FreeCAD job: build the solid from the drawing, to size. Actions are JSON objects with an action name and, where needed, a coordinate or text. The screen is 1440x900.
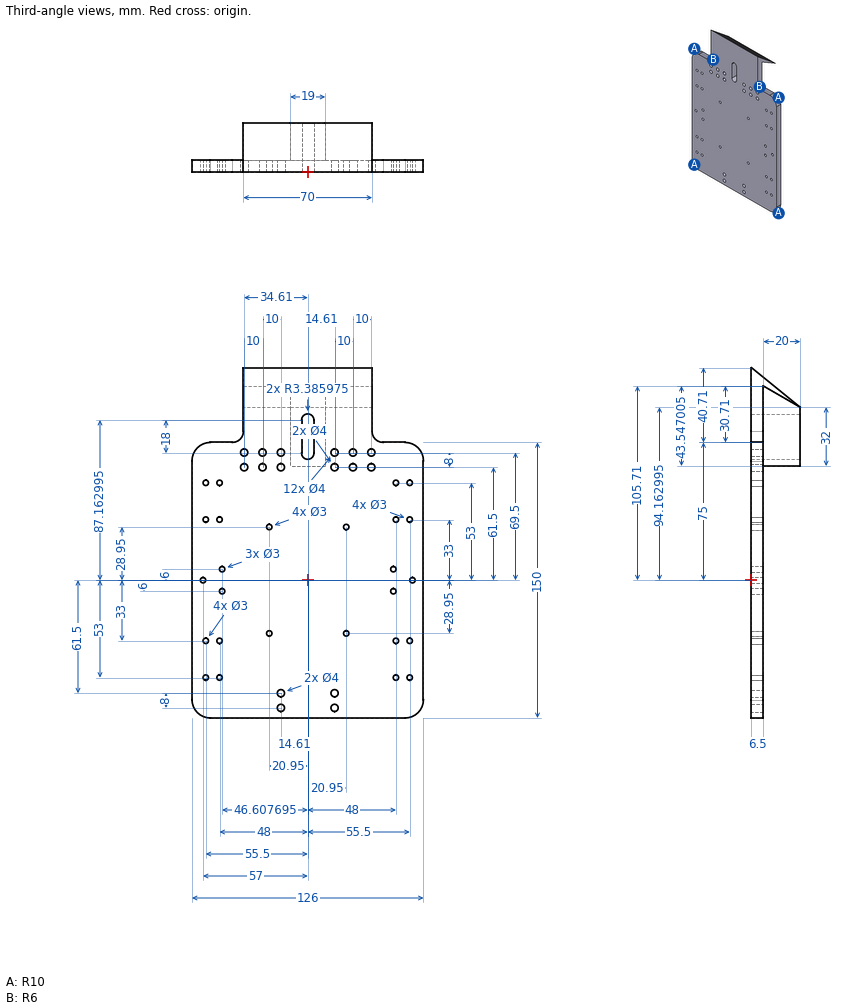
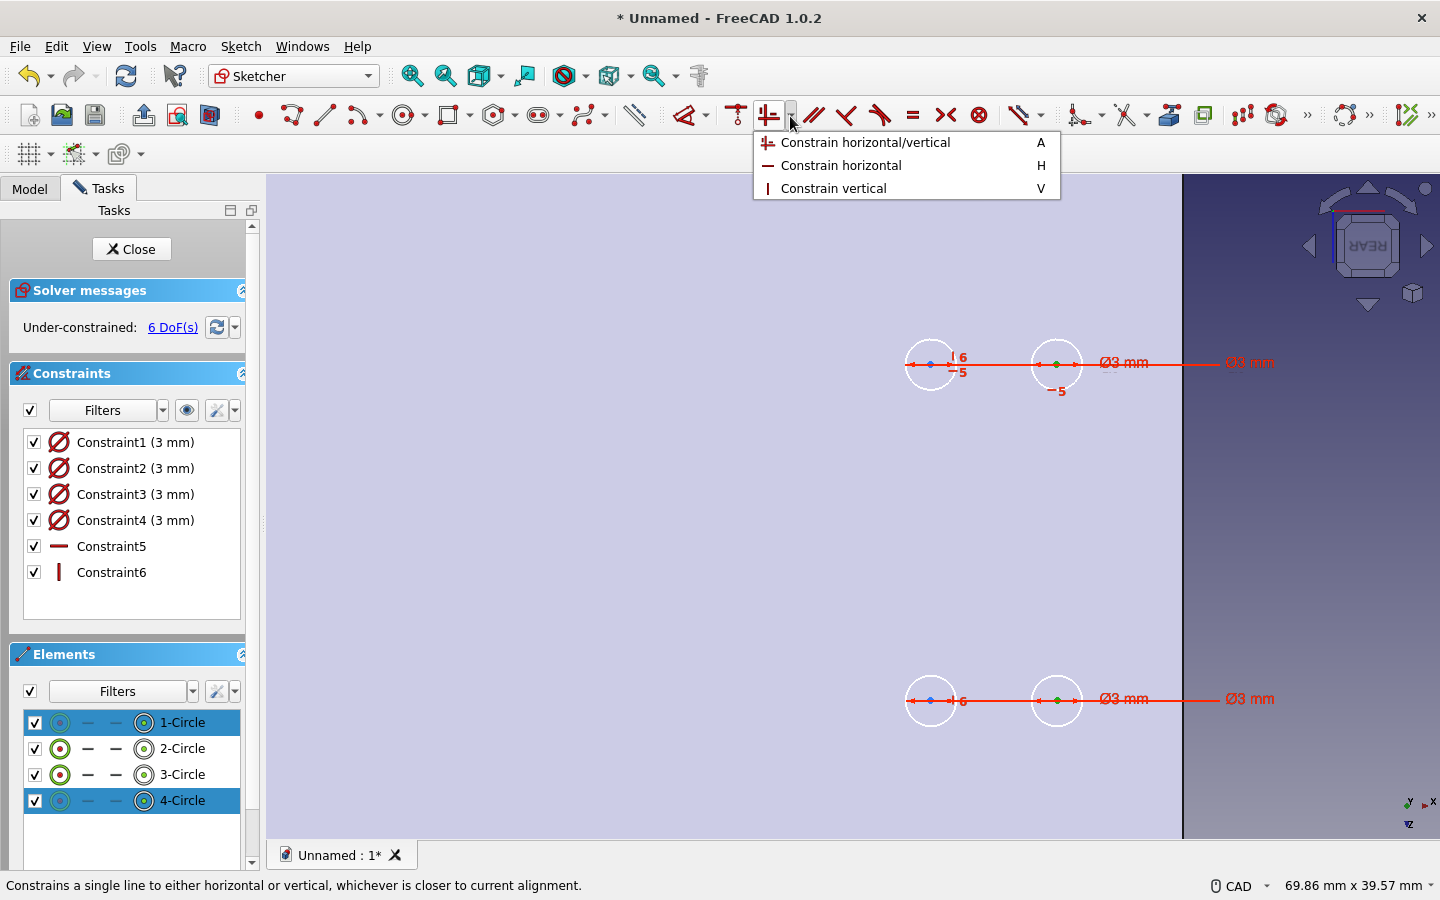
{"action": "left_click", "coordinate": [907, 188]}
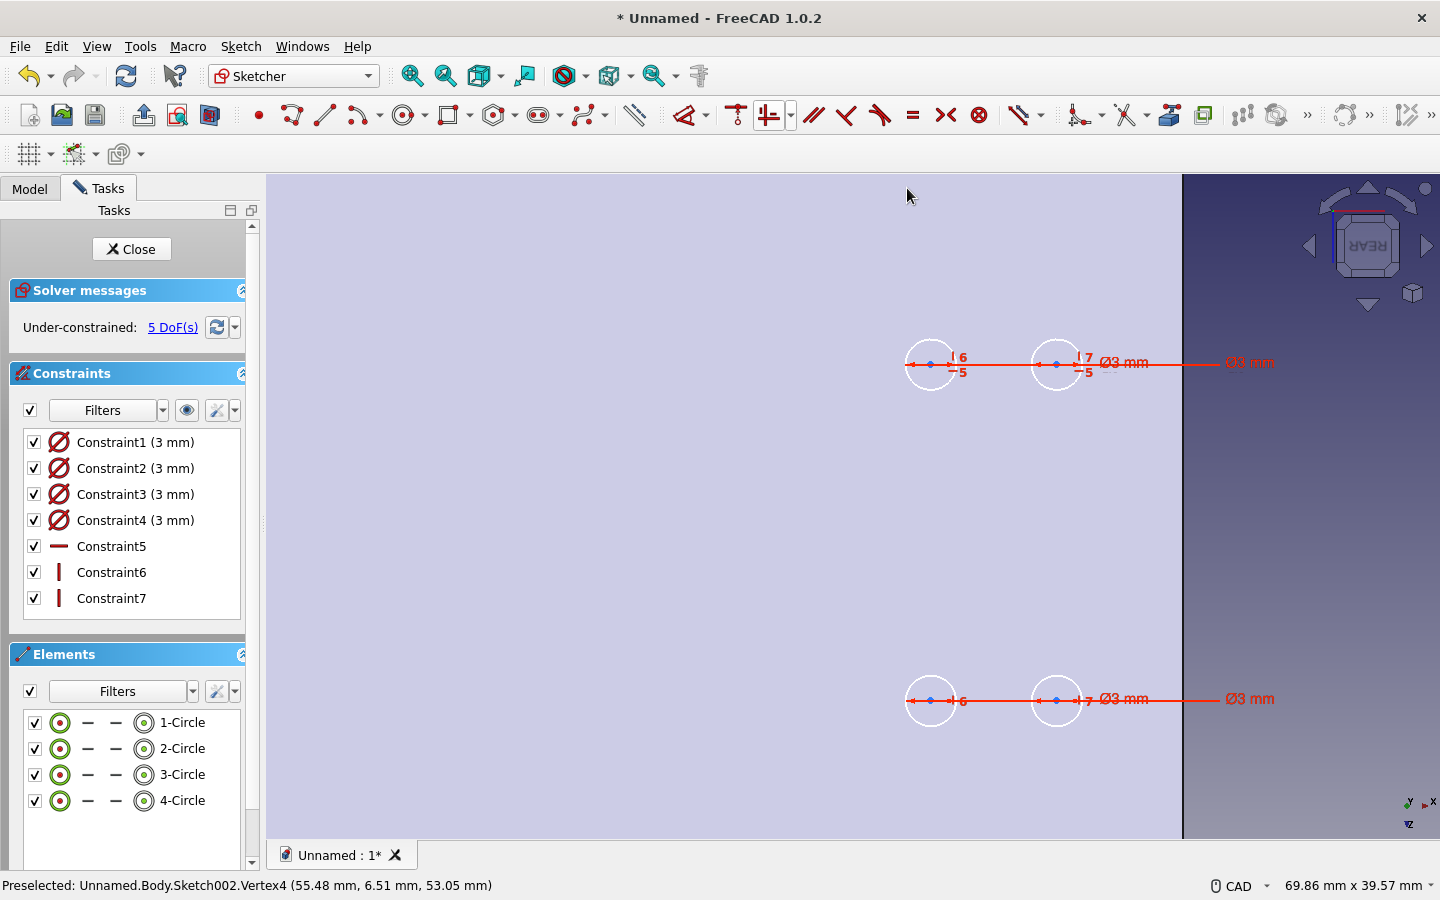
{"action": "left_click", "coordinate": [931, 701]}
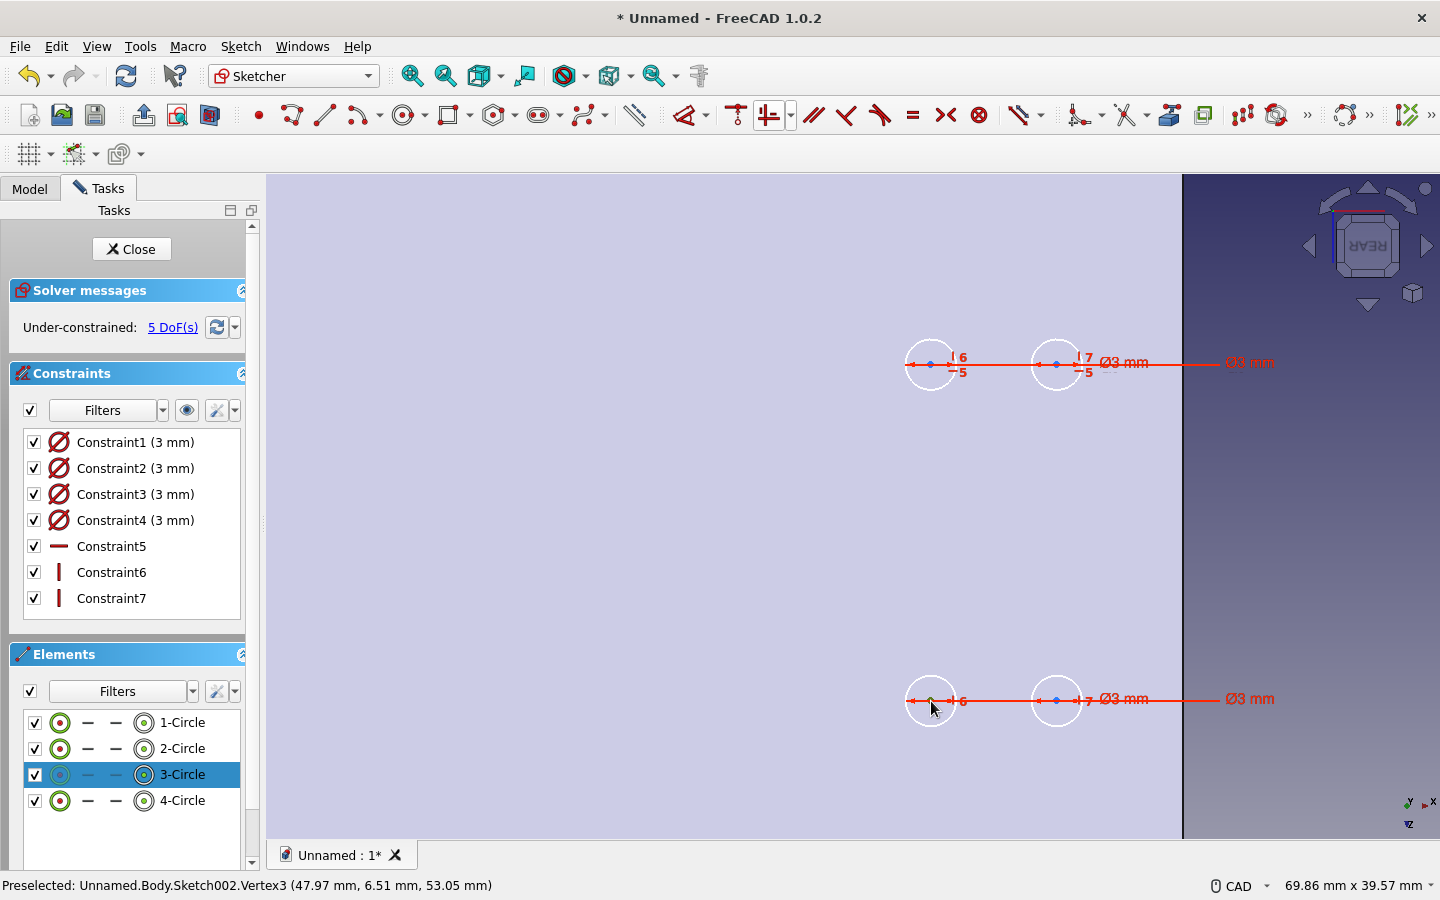
{"action": "left_click", "coordinate": [1057, 701]}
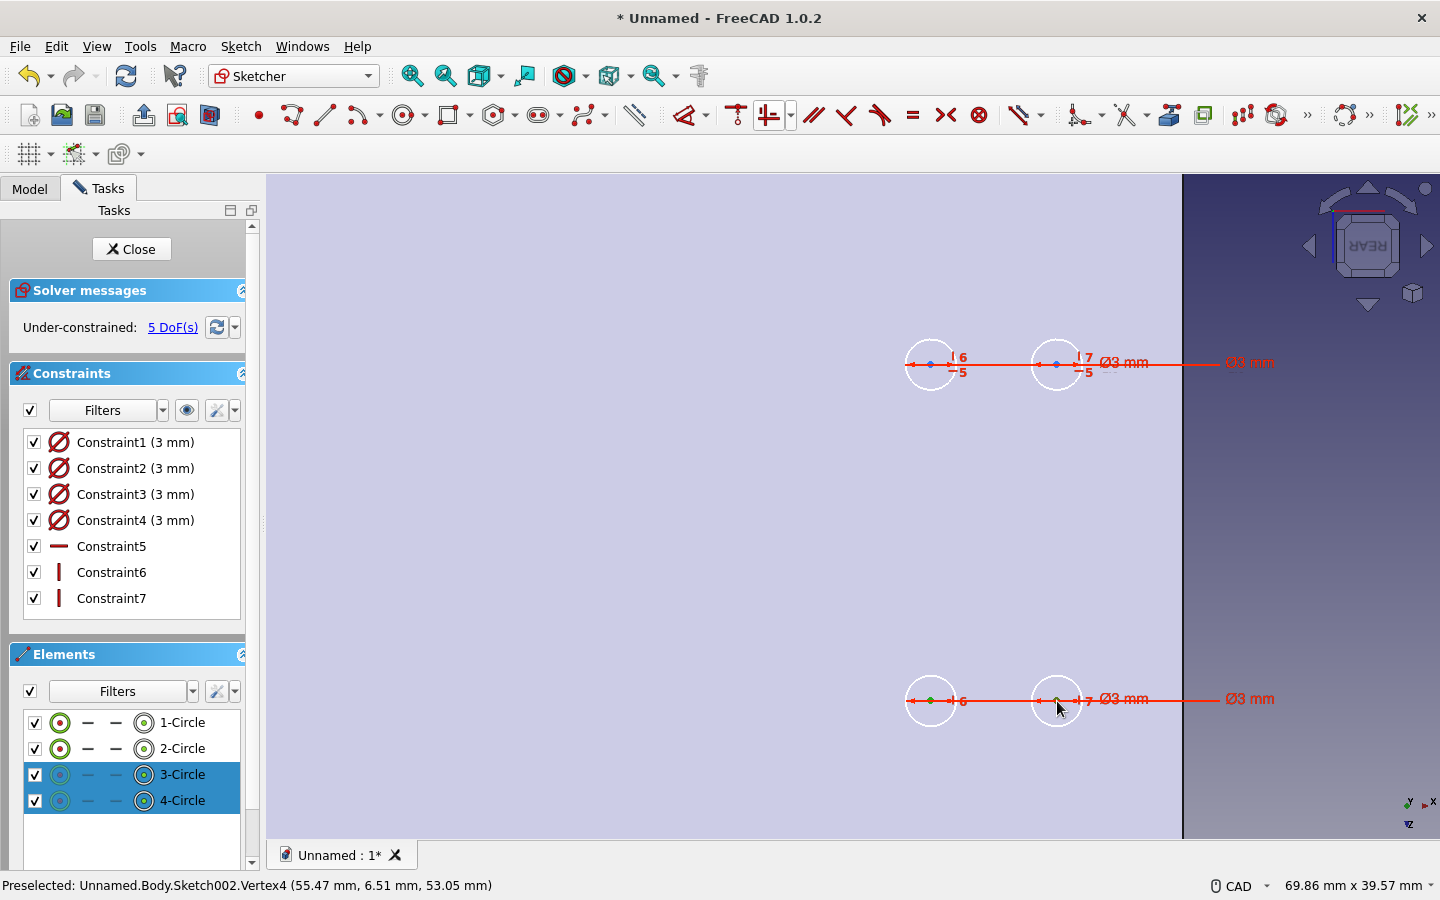
{"action": "key", "text": "h"}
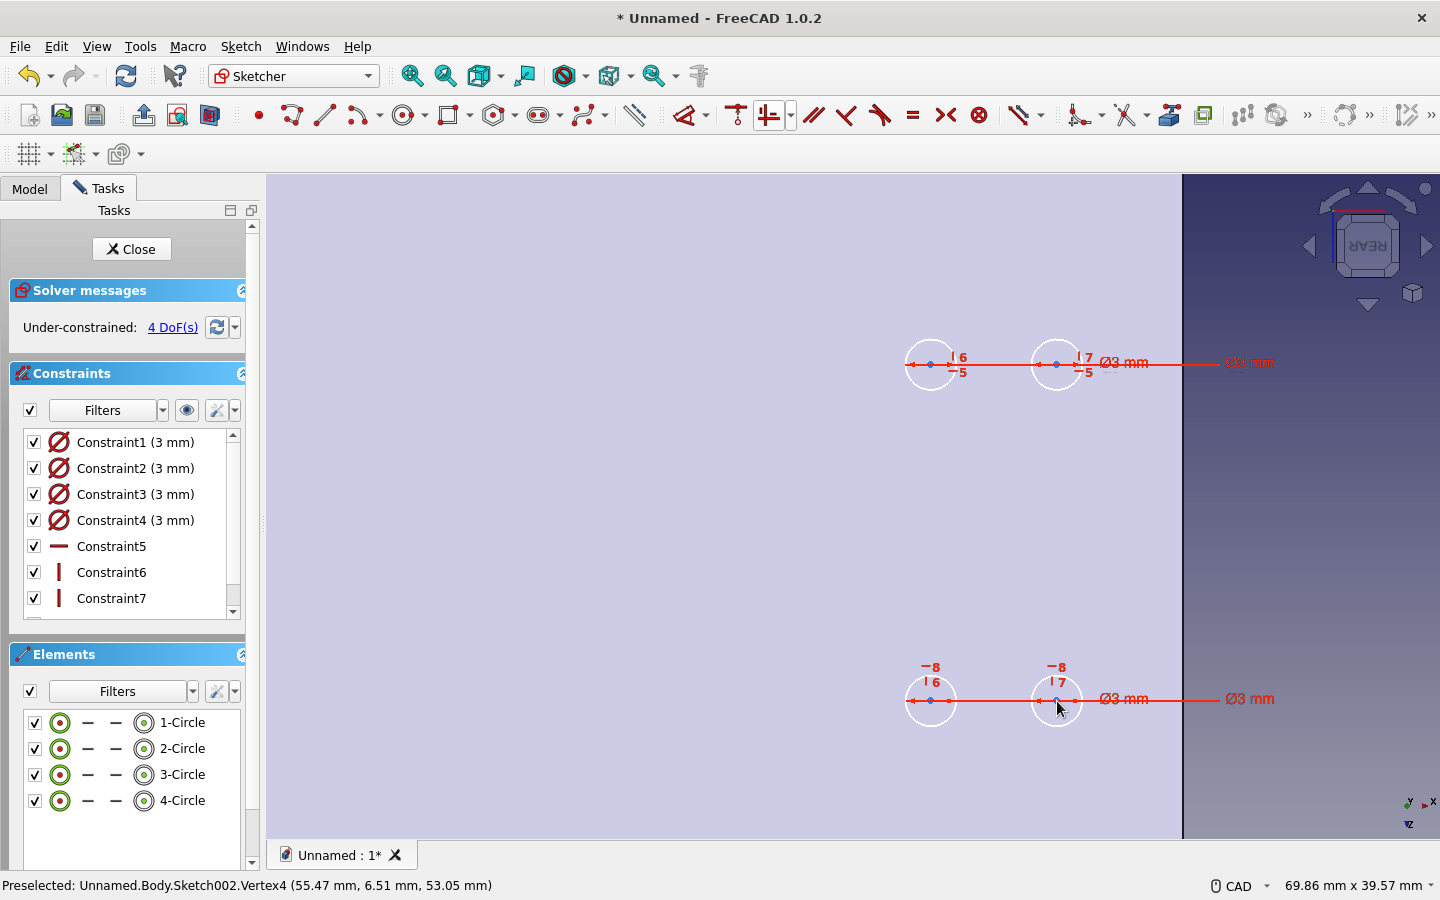
{"action": "key", "text": "d"}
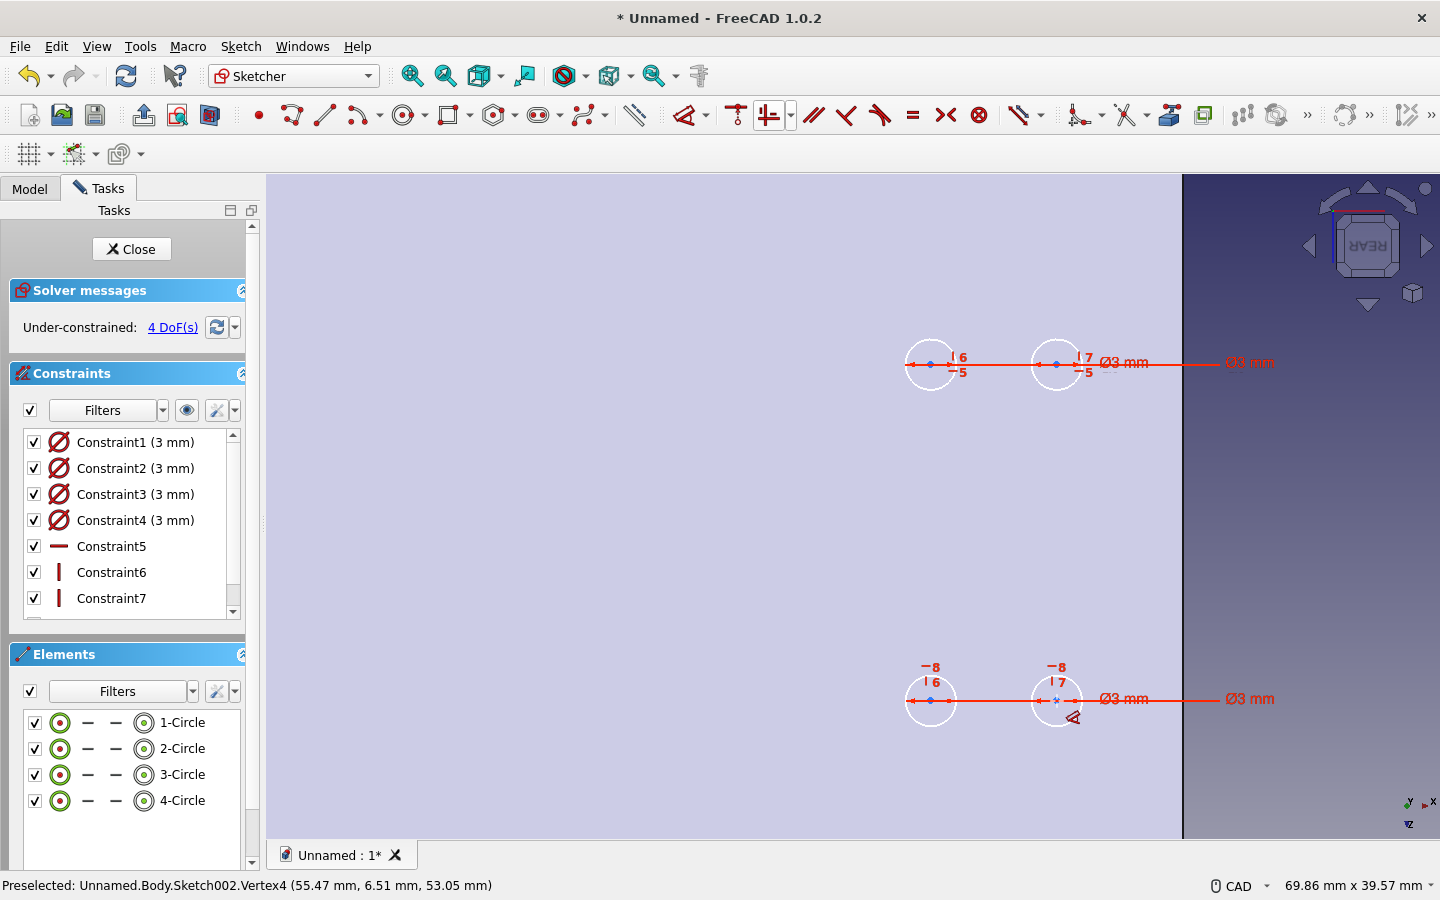
{"action": "left_click", "coordinate": [1057, 365]}
{"action": "left_click", "coordinate": [1091, 283]}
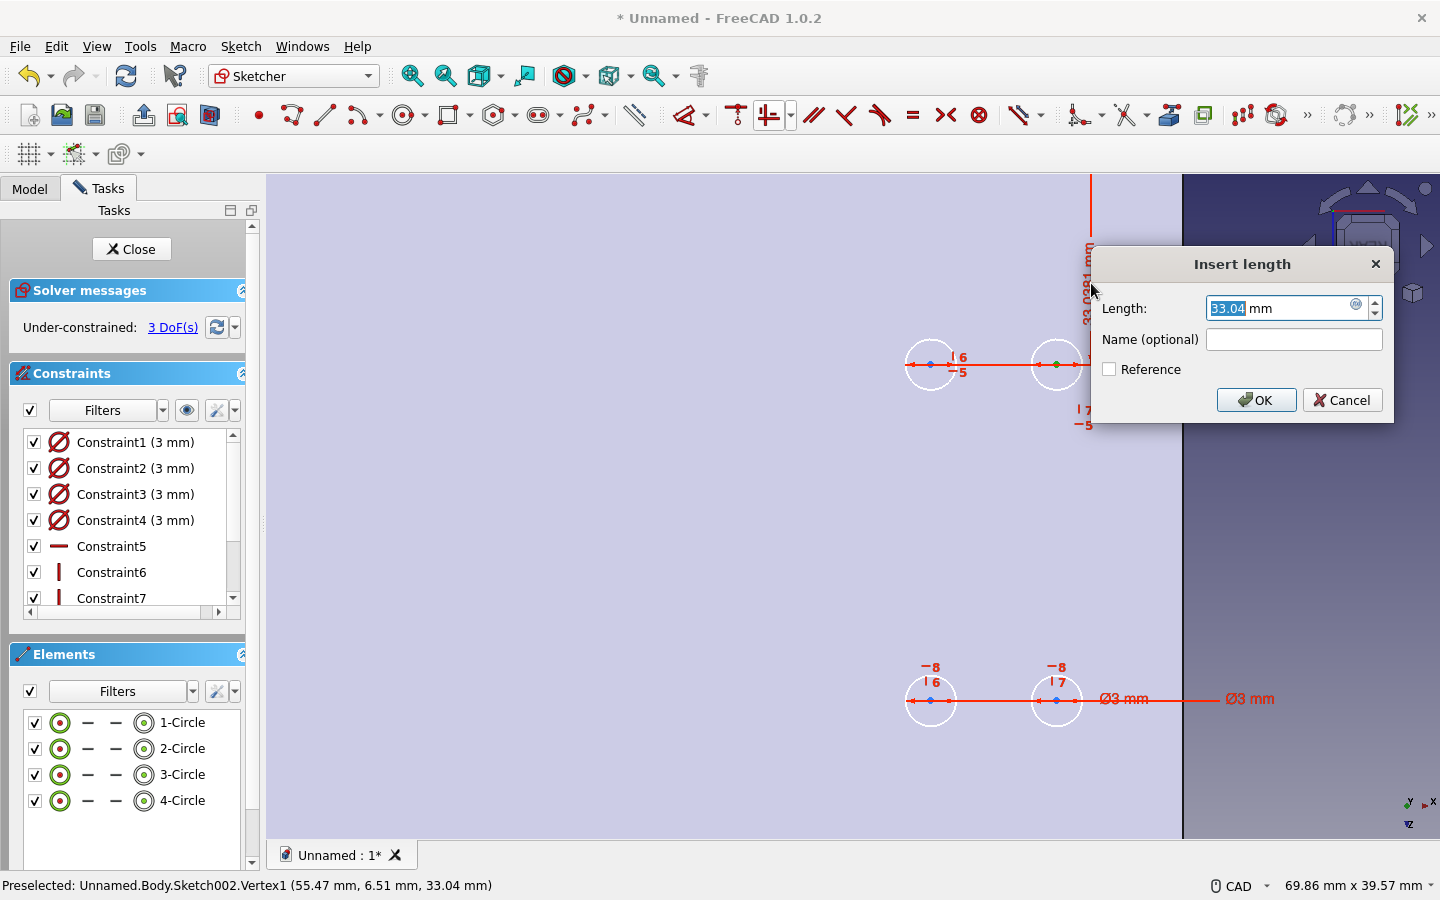
{"action": "type", "text": "33"}
{"action": "key", "text": "Return"}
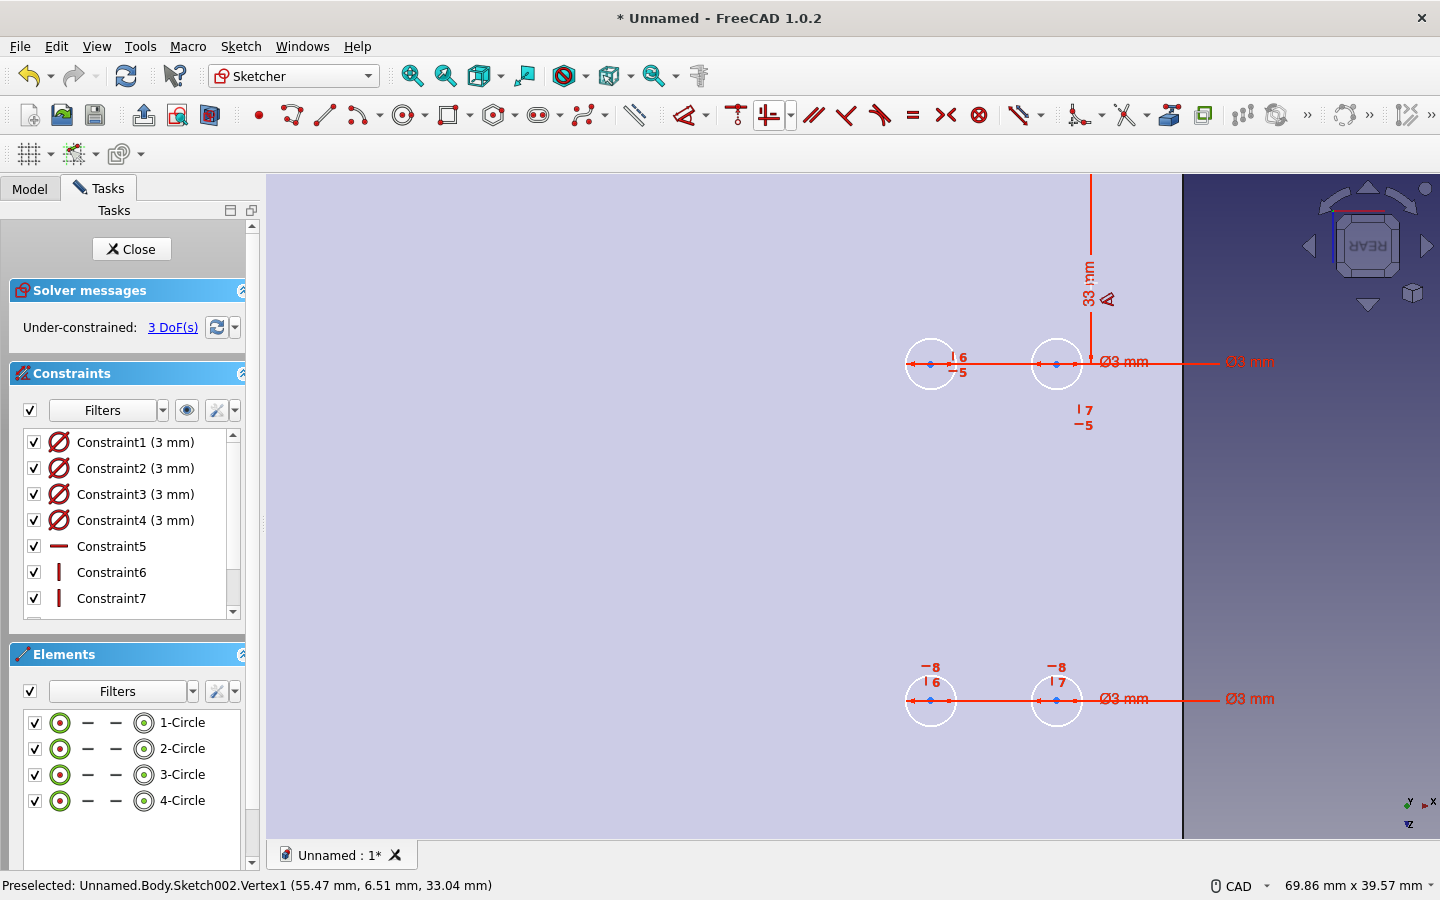
{"action": "left_click", "coordinate": [931, 364]}
{"action": "left_click", "coordinate": [612, 398]}